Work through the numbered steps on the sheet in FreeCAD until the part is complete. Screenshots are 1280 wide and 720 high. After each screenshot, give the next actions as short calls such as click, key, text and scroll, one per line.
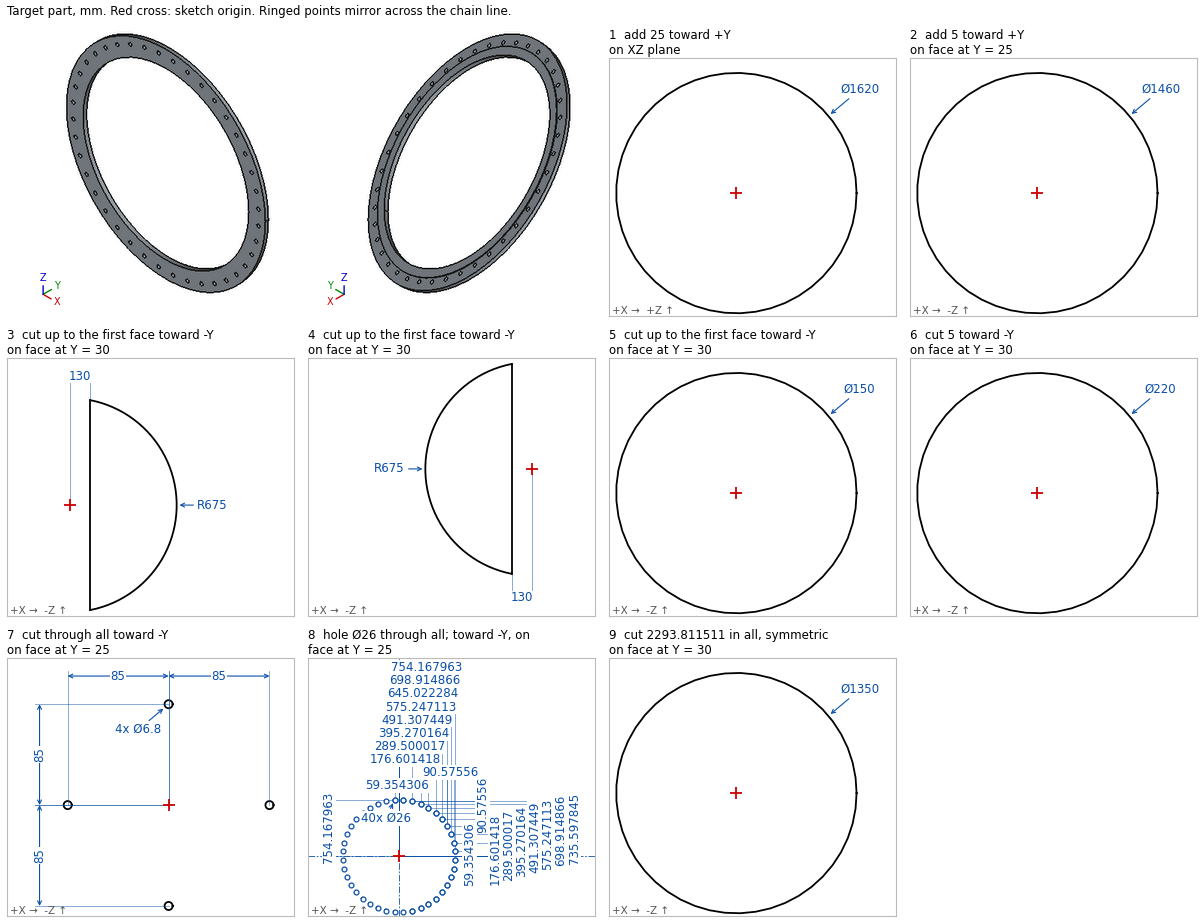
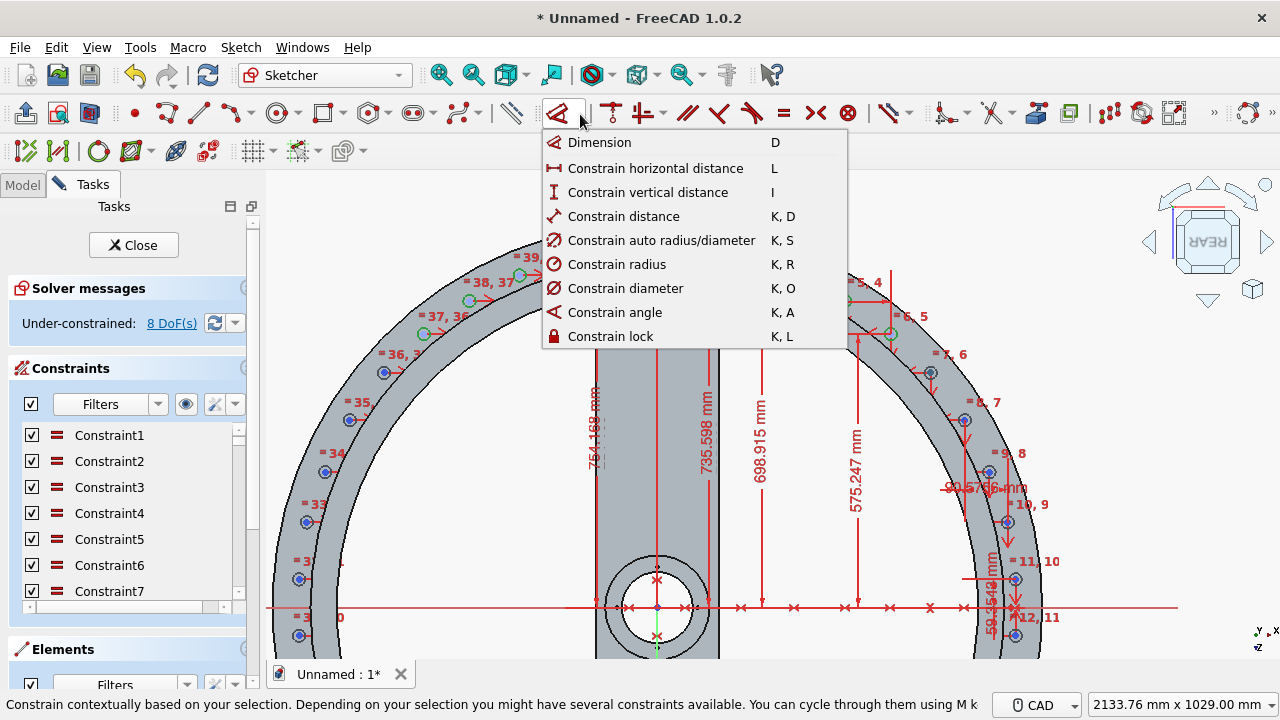
click(695, 168)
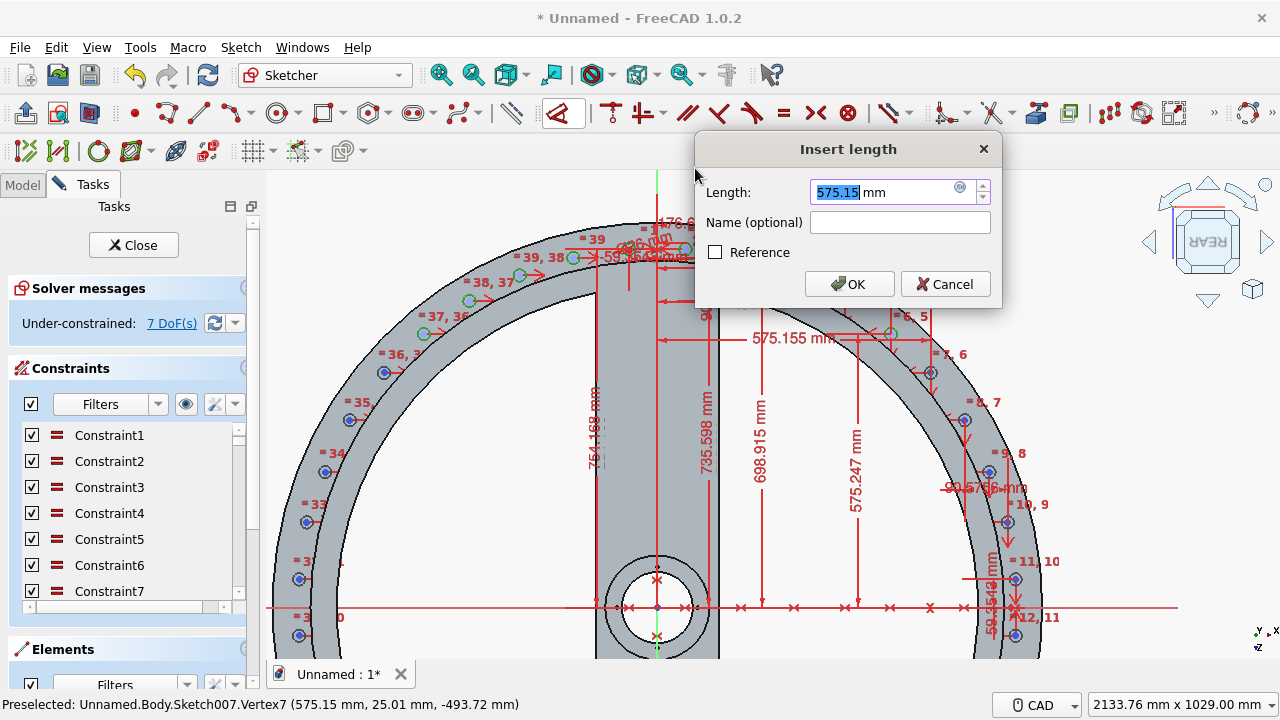
text(575.247113)
key(Return)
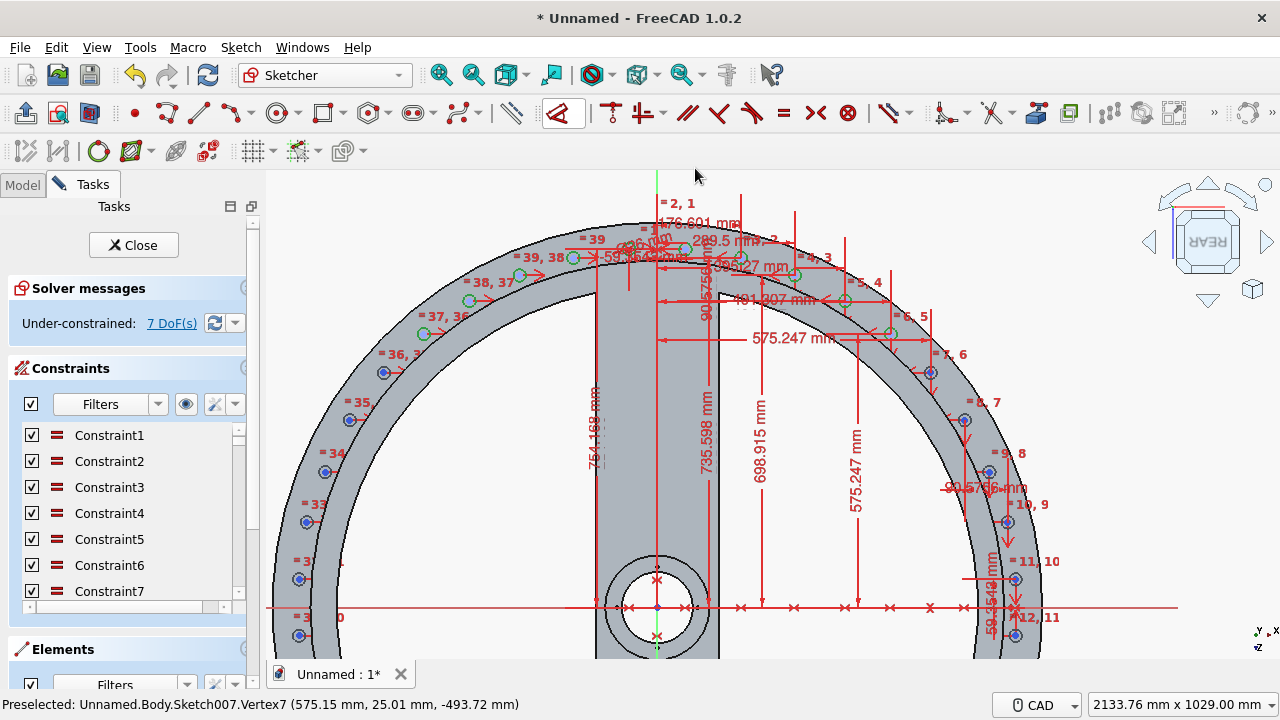
click(931, 373)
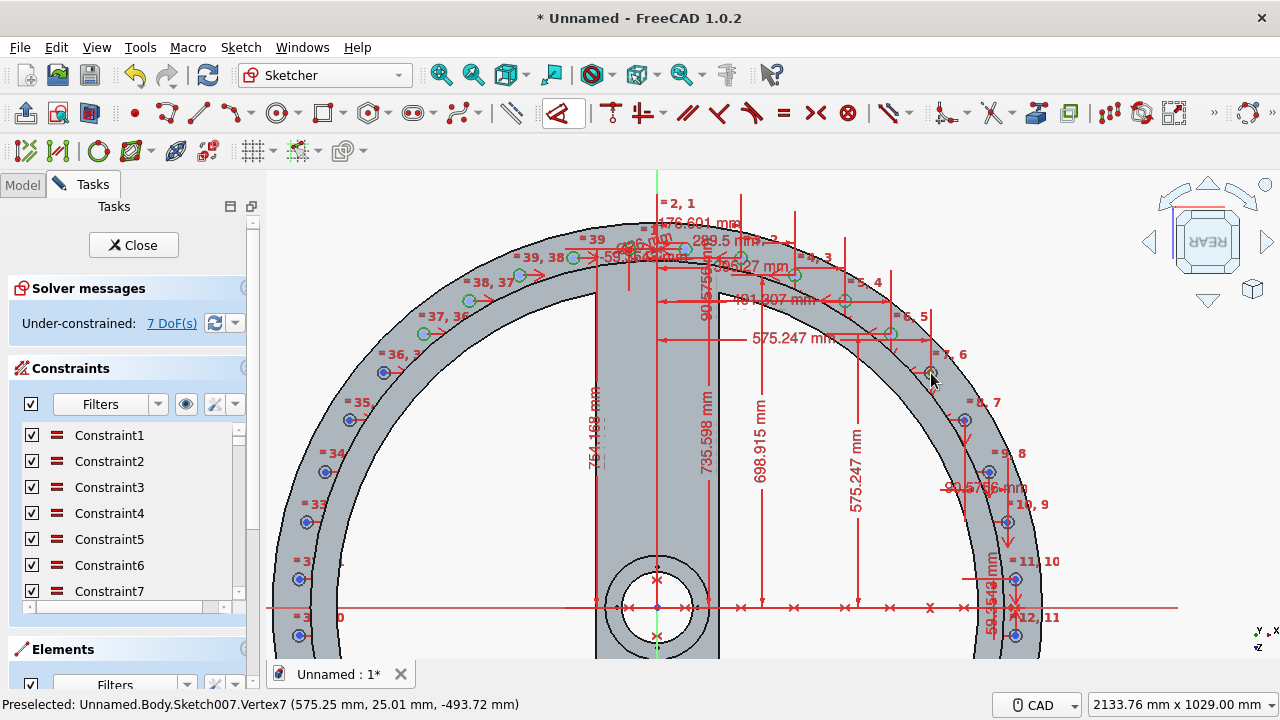
click(580, 114)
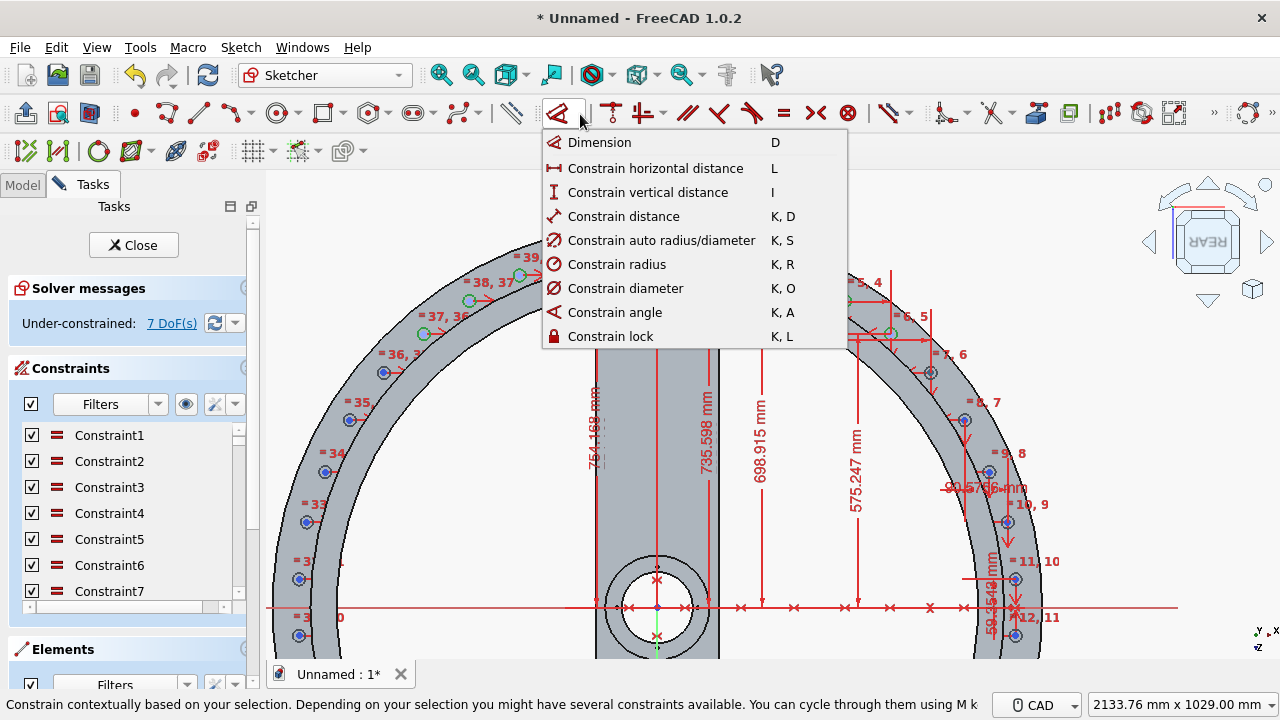
click(695, 192)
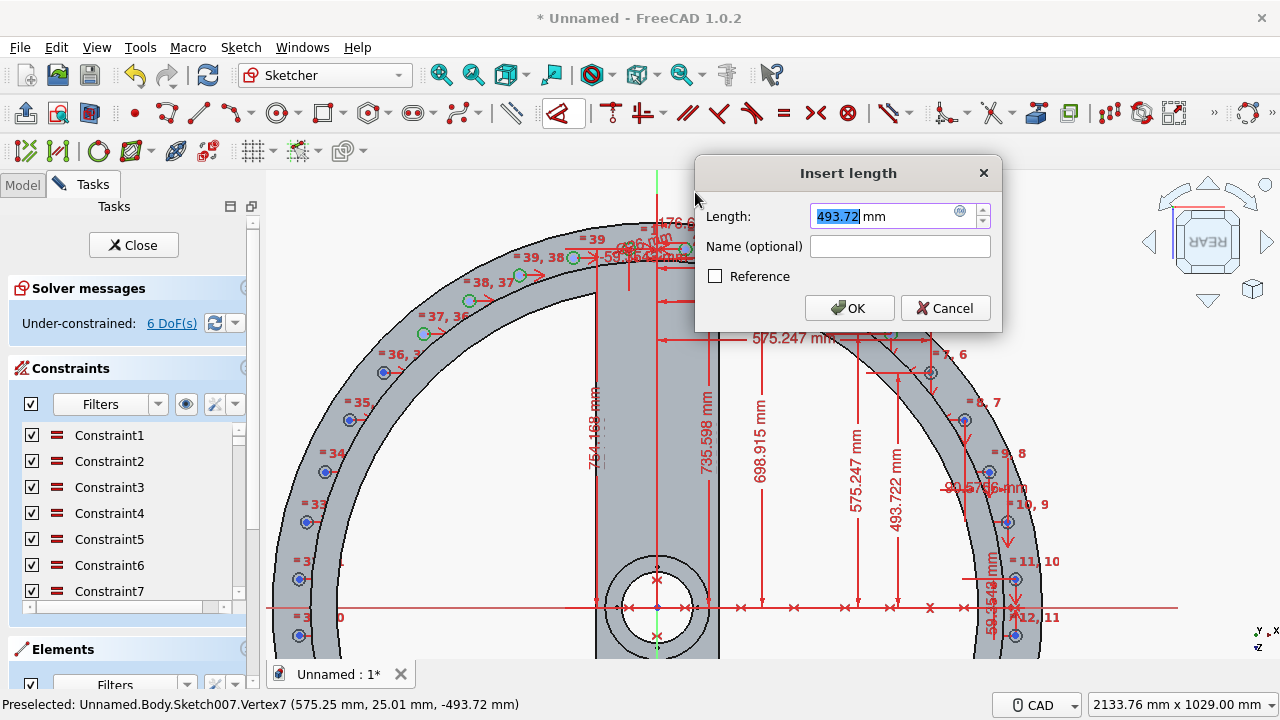
text(491.307449)
key(Return)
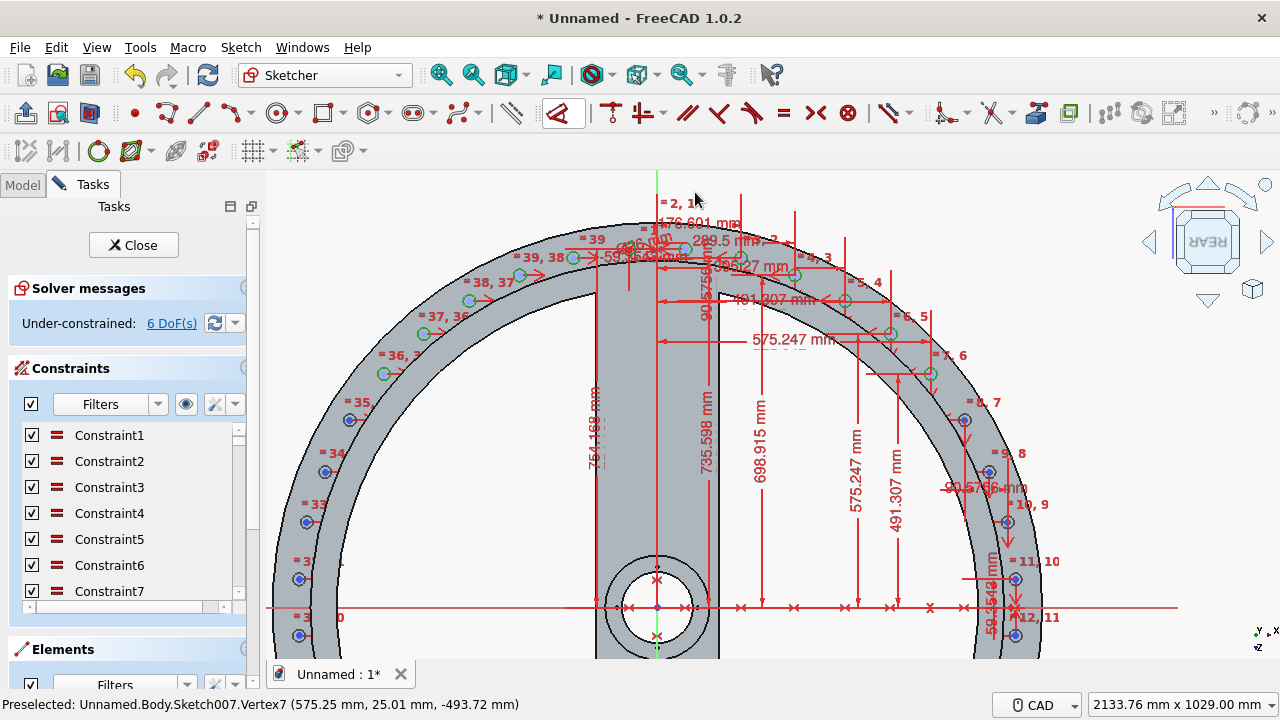
click(965, 420)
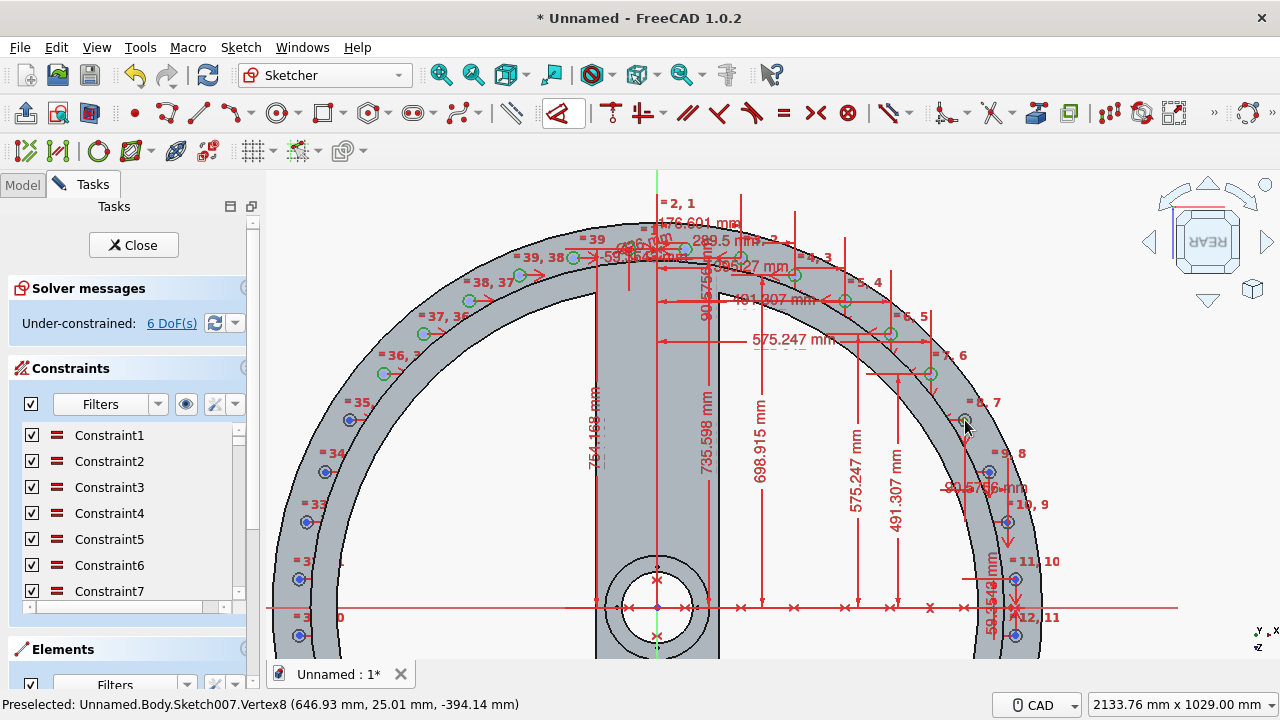
click(580, 114)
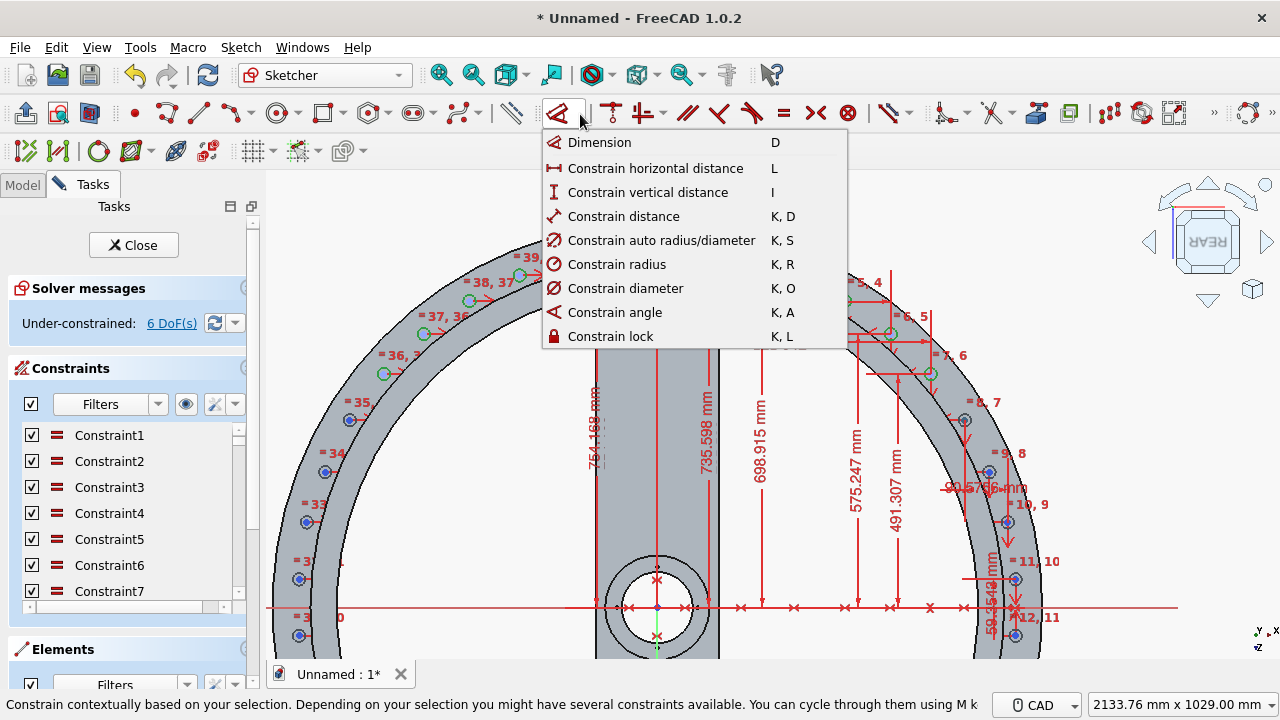
click(695, 168)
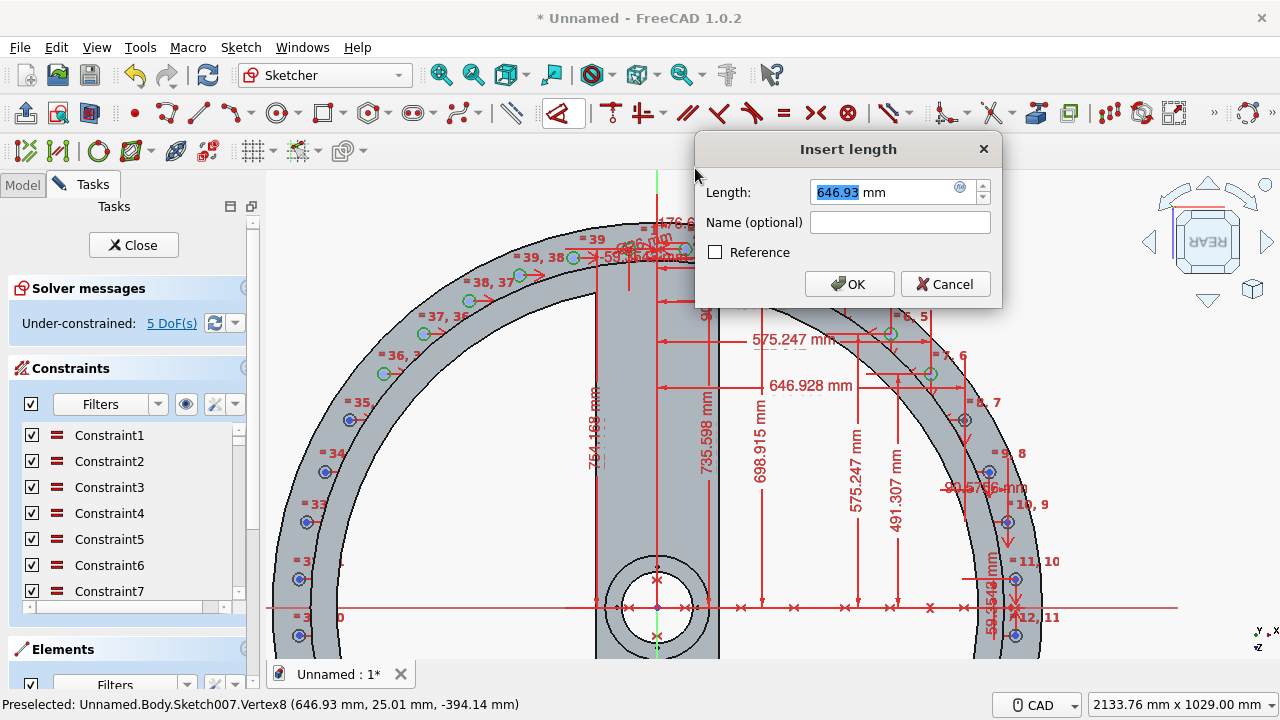
text(645.022284)
key(Return)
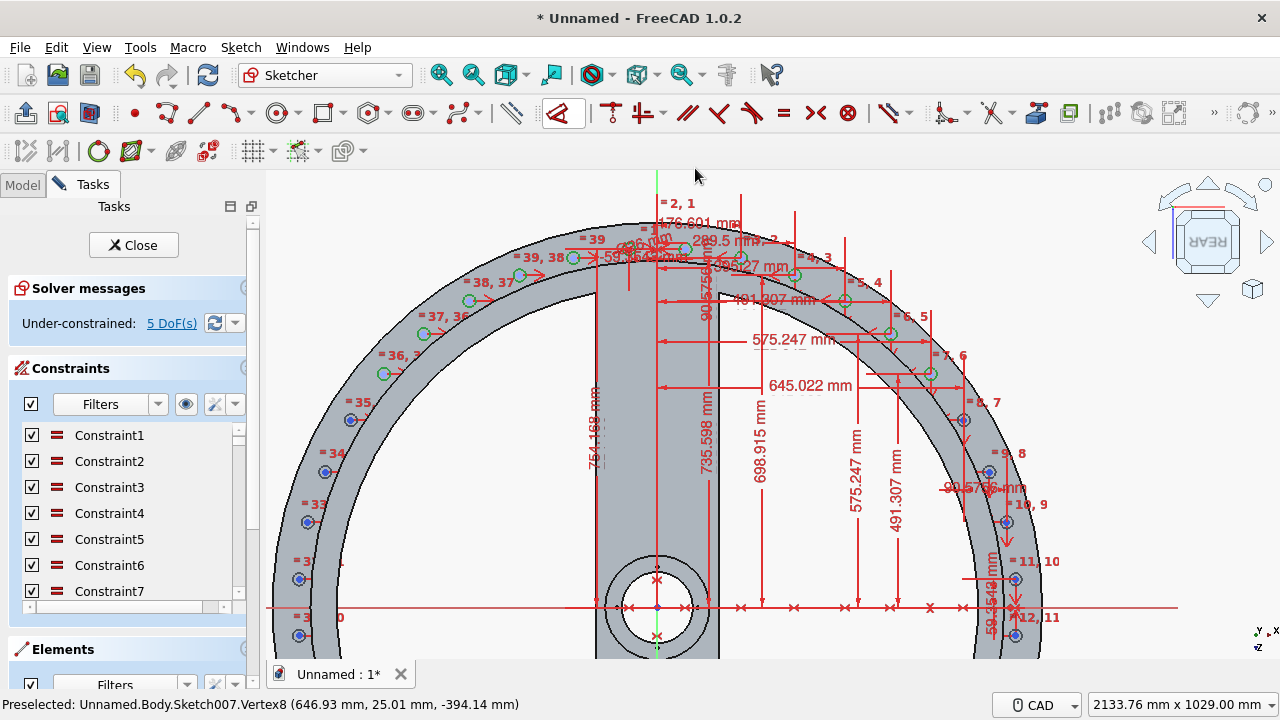
click(964, 420)